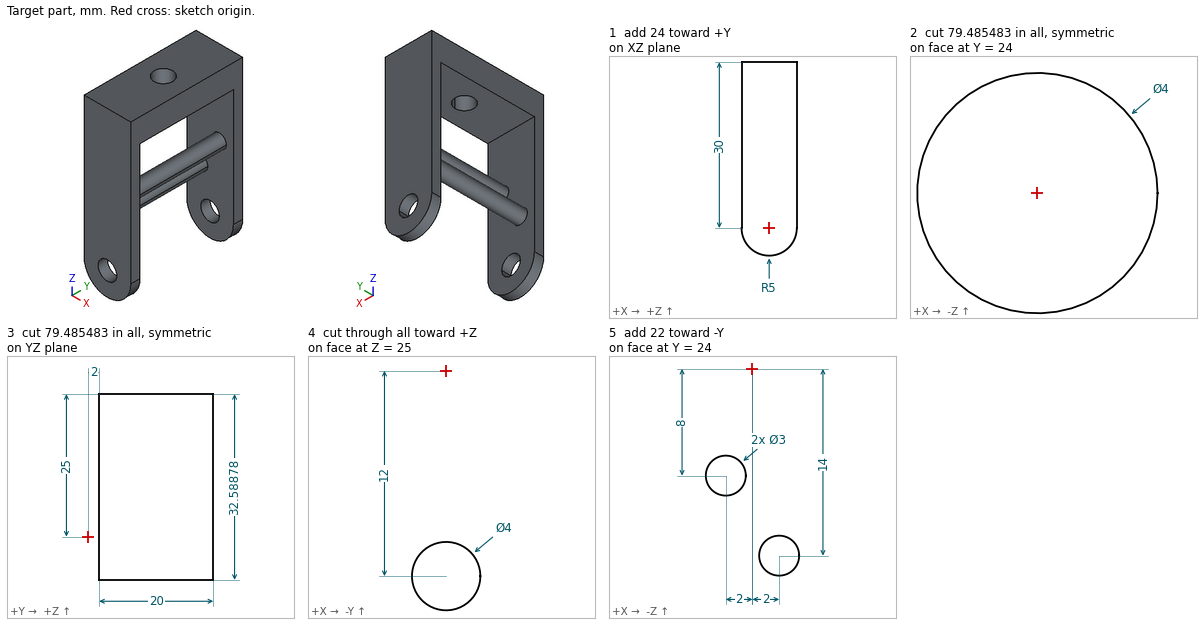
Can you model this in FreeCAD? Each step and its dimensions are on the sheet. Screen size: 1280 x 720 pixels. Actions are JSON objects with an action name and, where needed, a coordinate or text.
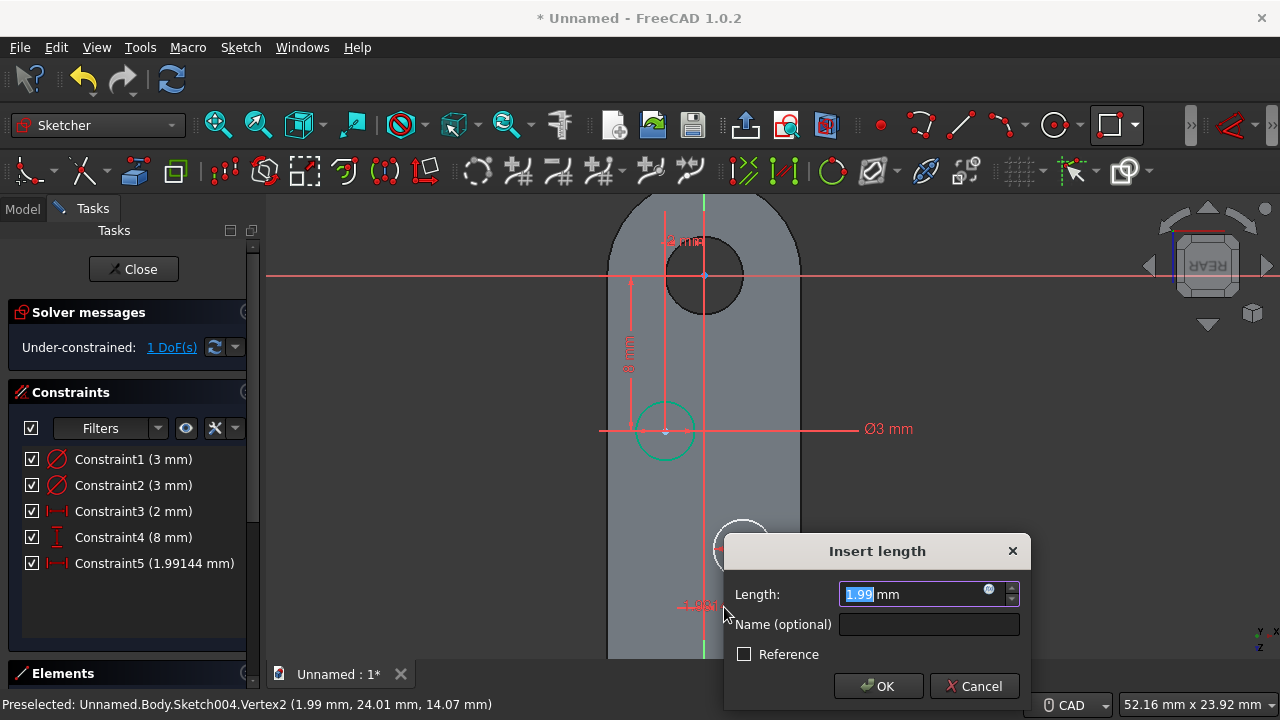
{"action": "type", "text": "2"}
{"action": "key", "text": "Return"}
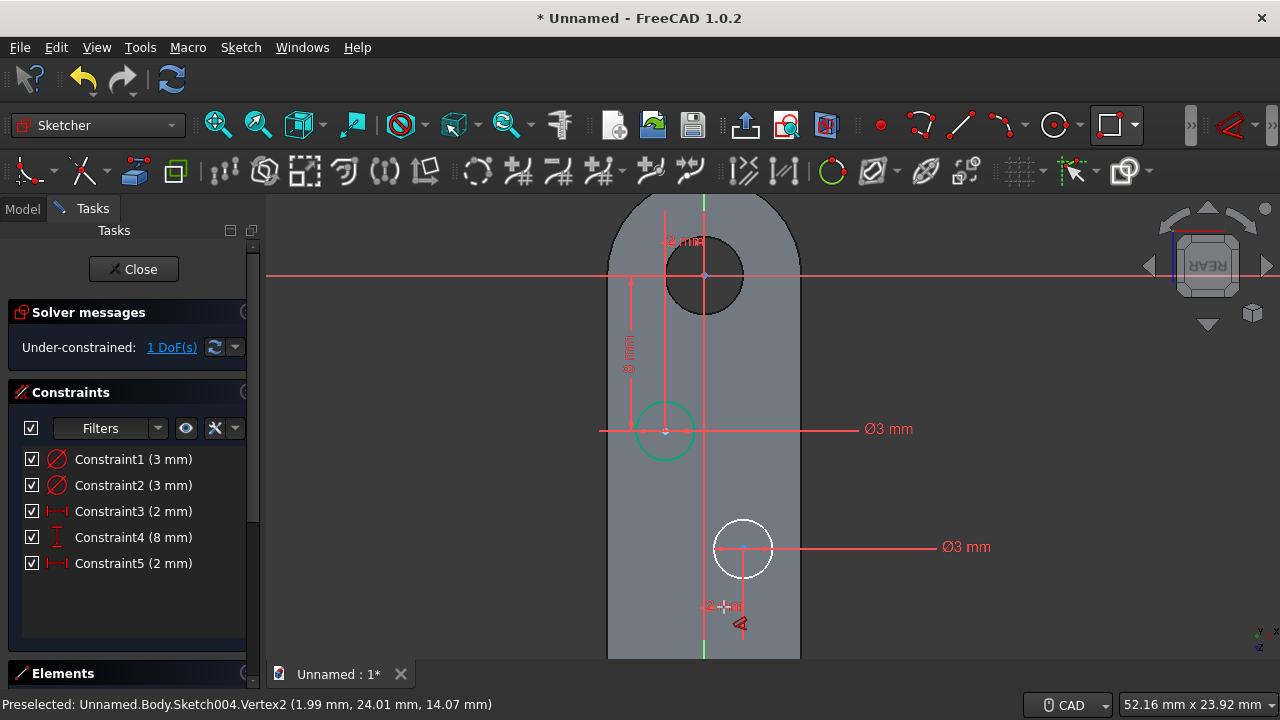
{"action": "left_click", "coordinate": [743, 549]}
{"action": "left_click", "coordinate": [777, 412]}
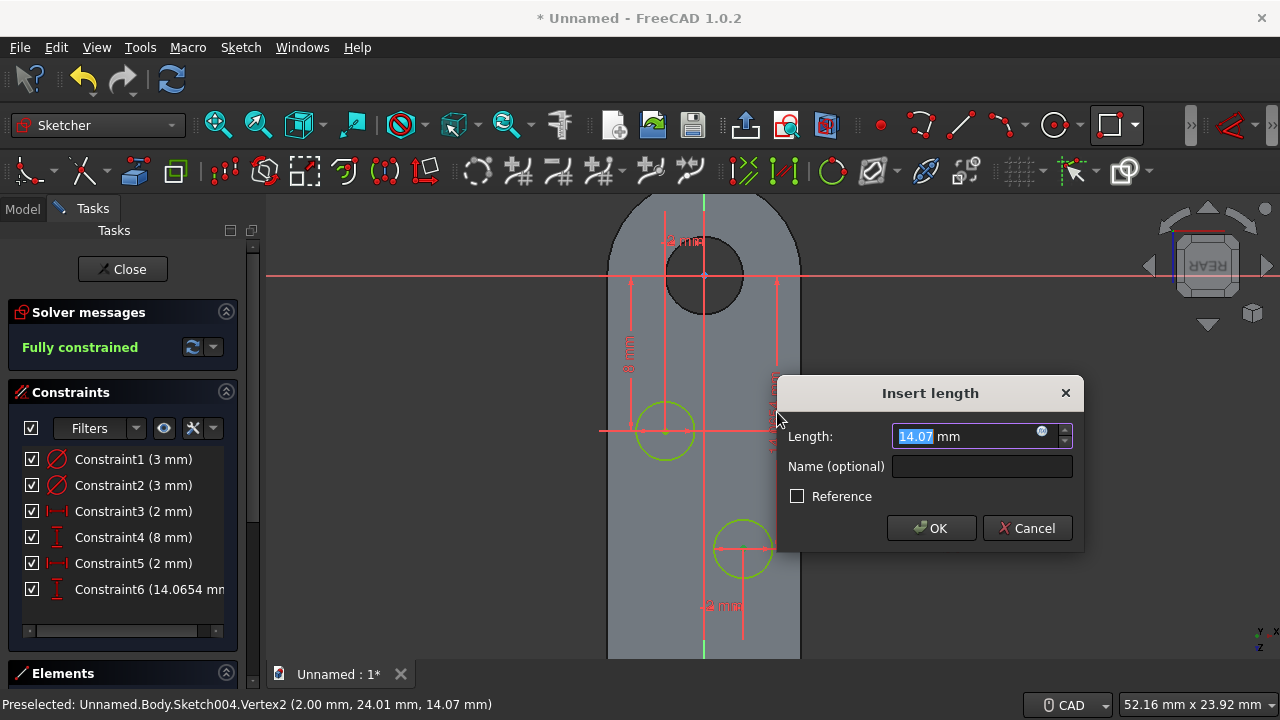
{"action": "type", "text": "14"}
{"action": "key", "text": "Return"}
{"action": "key", "text": "Escape"}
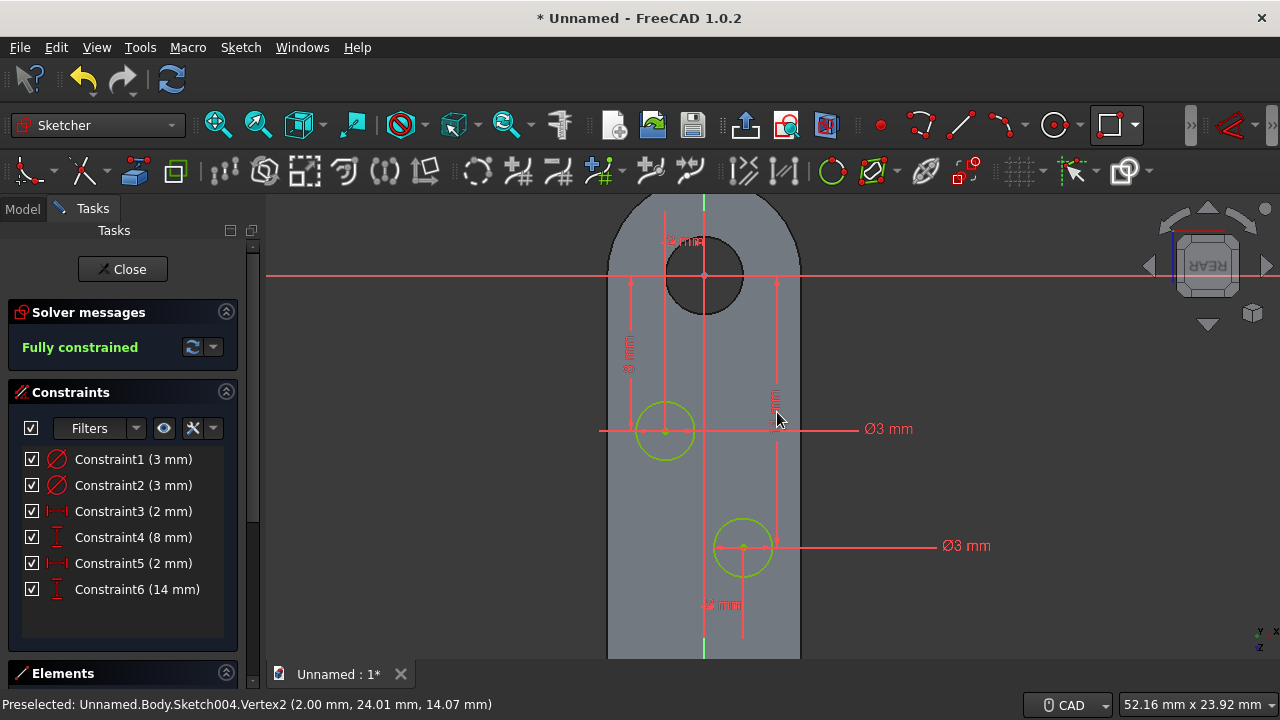
{"action": "left_click", "coordinate": [123, 269]}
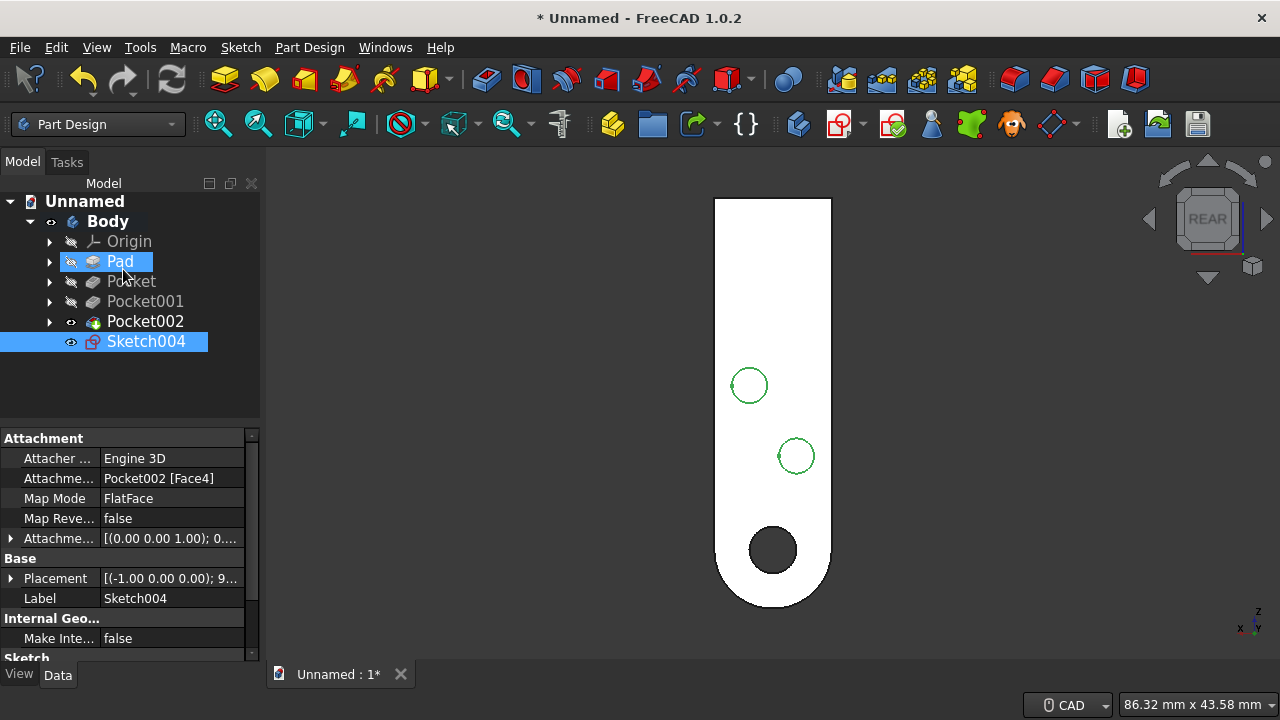
{"action": "left_click", "coordinate": [226, 80]}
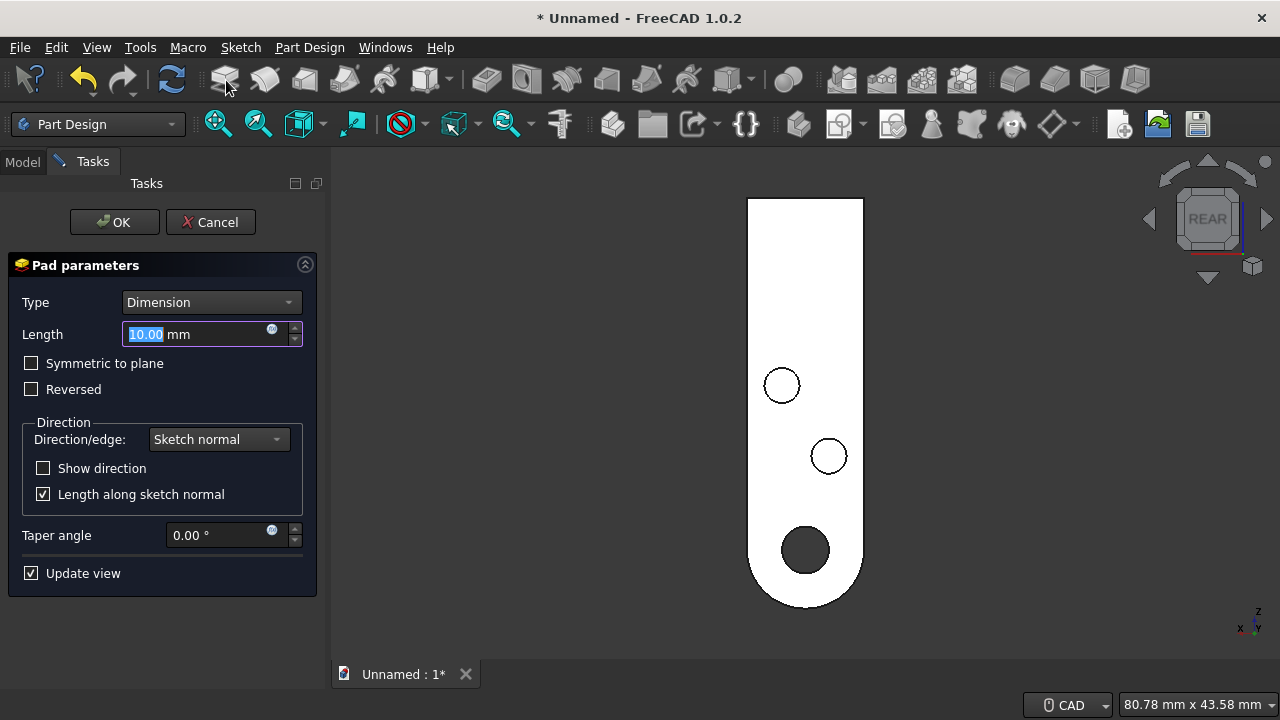
{"action": "type", "text": "22"}
{"action": "key", "text": "Tab"}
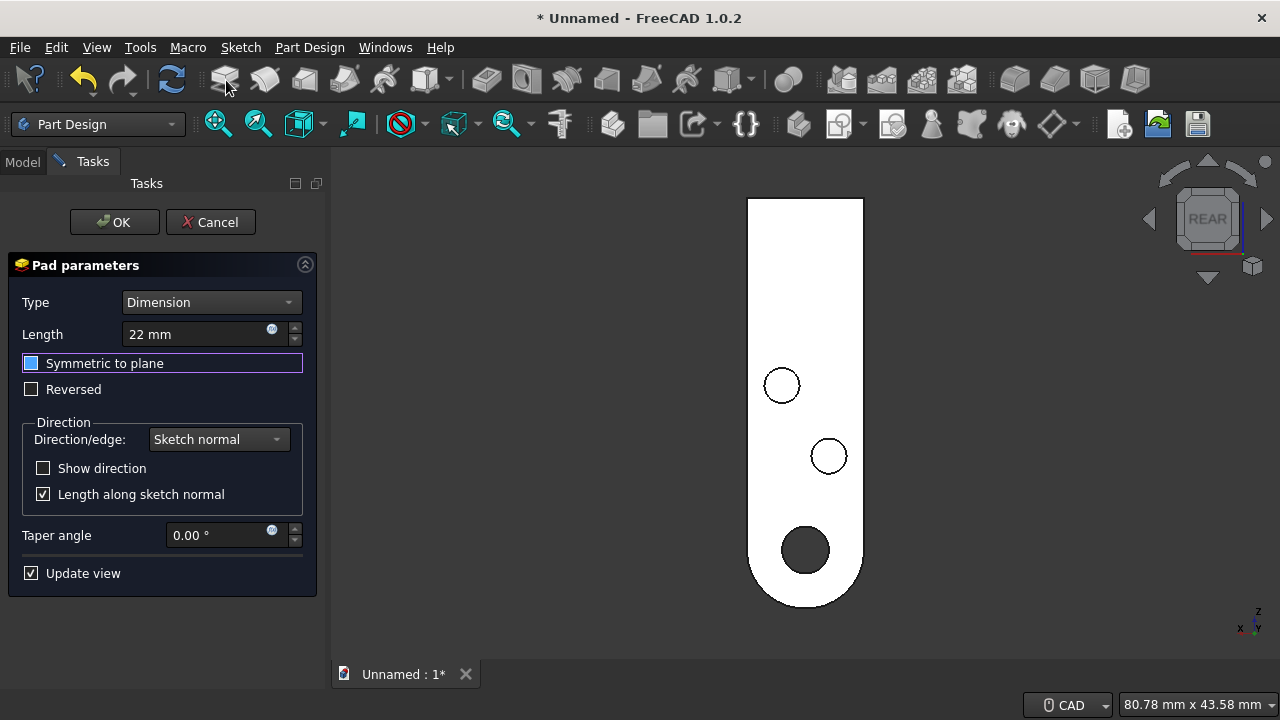
{"action": "left_click", "coordinate": [30, 389]}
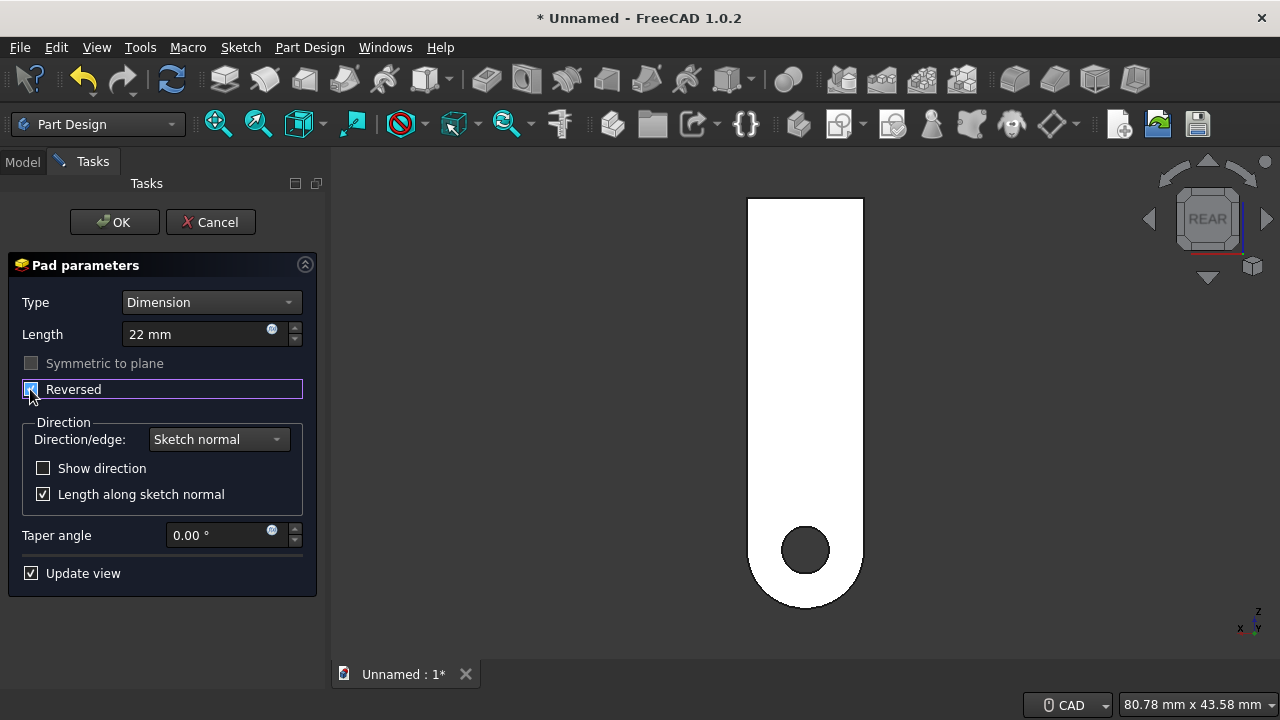
{"action": "left_click", "coordinate": [115, 222]}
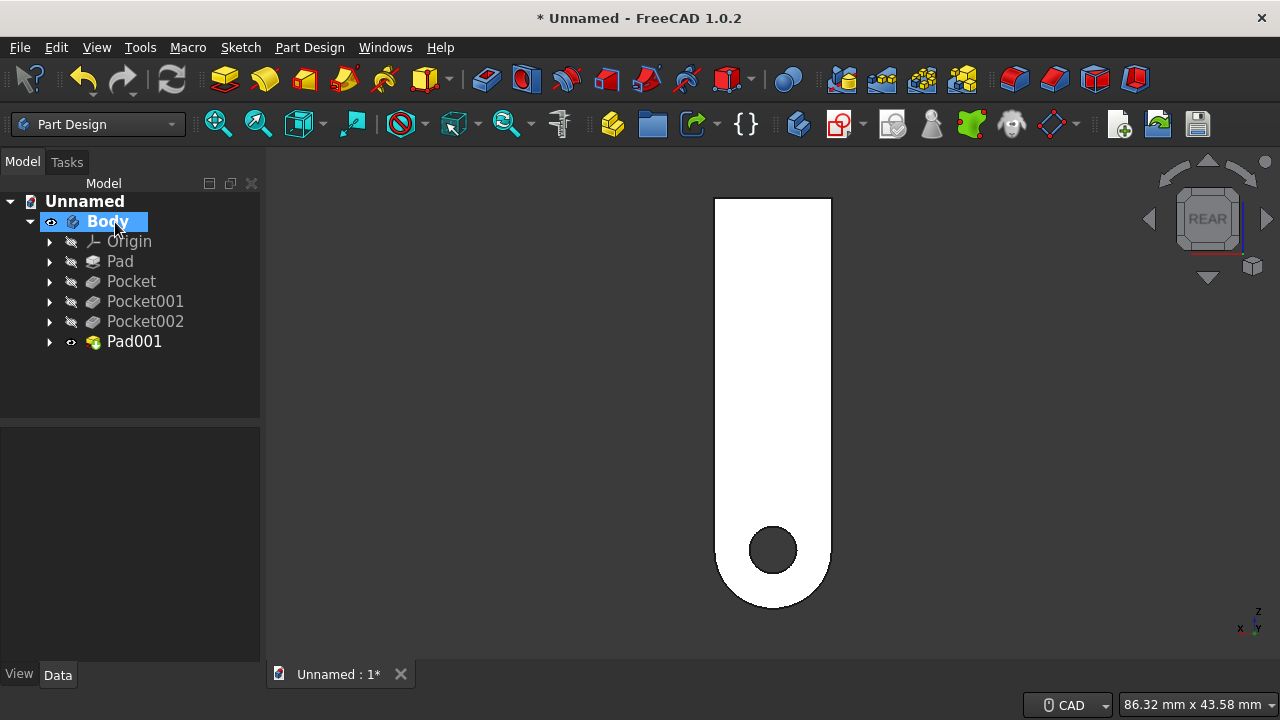
{"action": "key", "text": "0"}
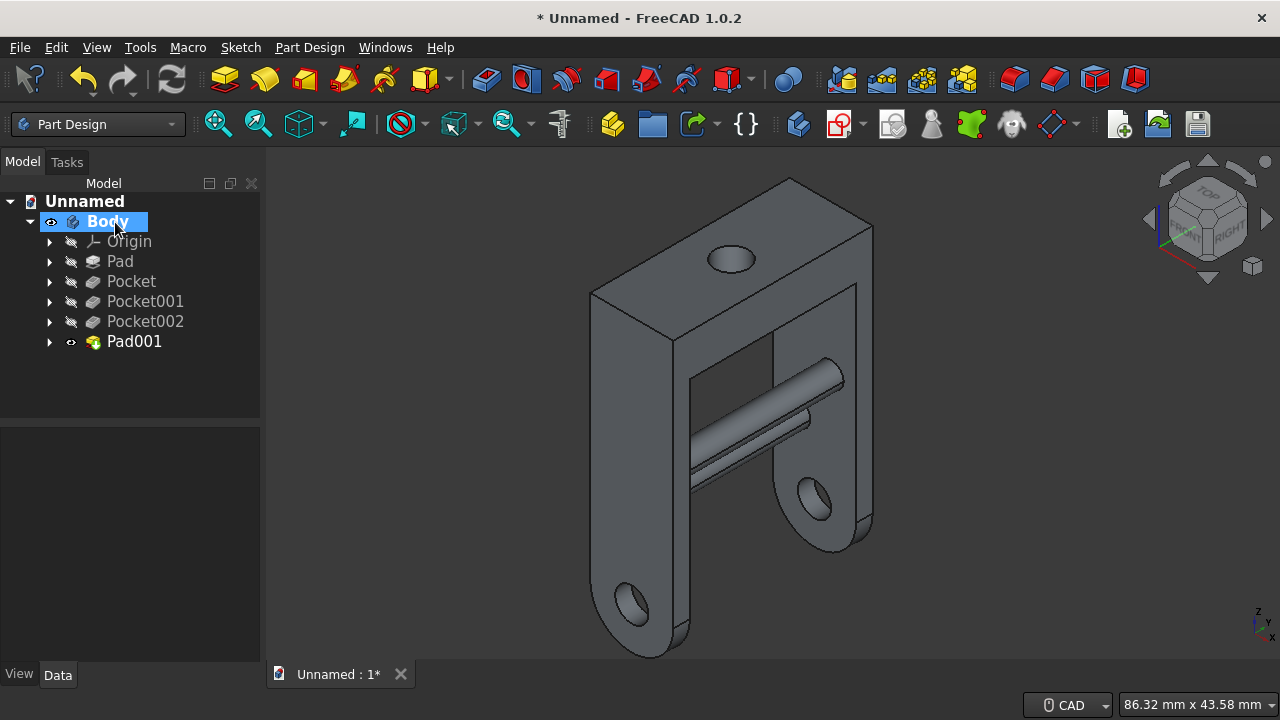
{"action": "left_click", "coordinate": [220, 124]}